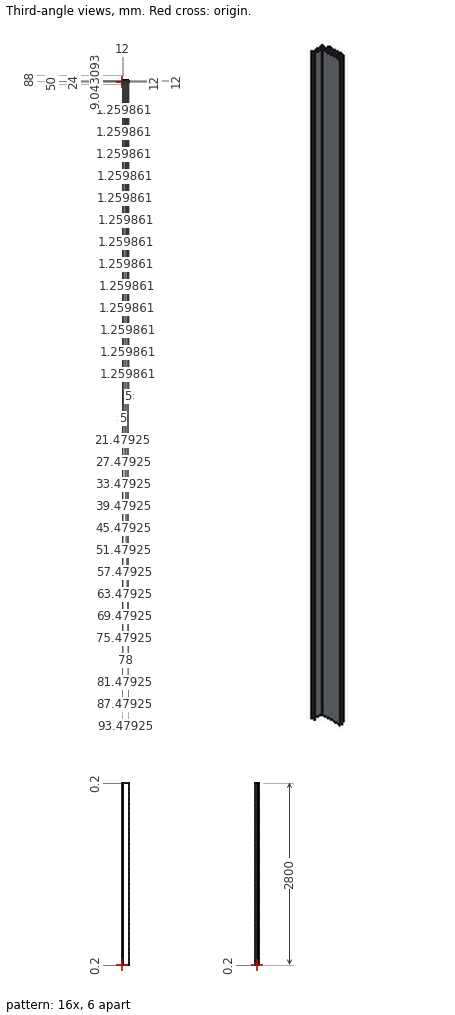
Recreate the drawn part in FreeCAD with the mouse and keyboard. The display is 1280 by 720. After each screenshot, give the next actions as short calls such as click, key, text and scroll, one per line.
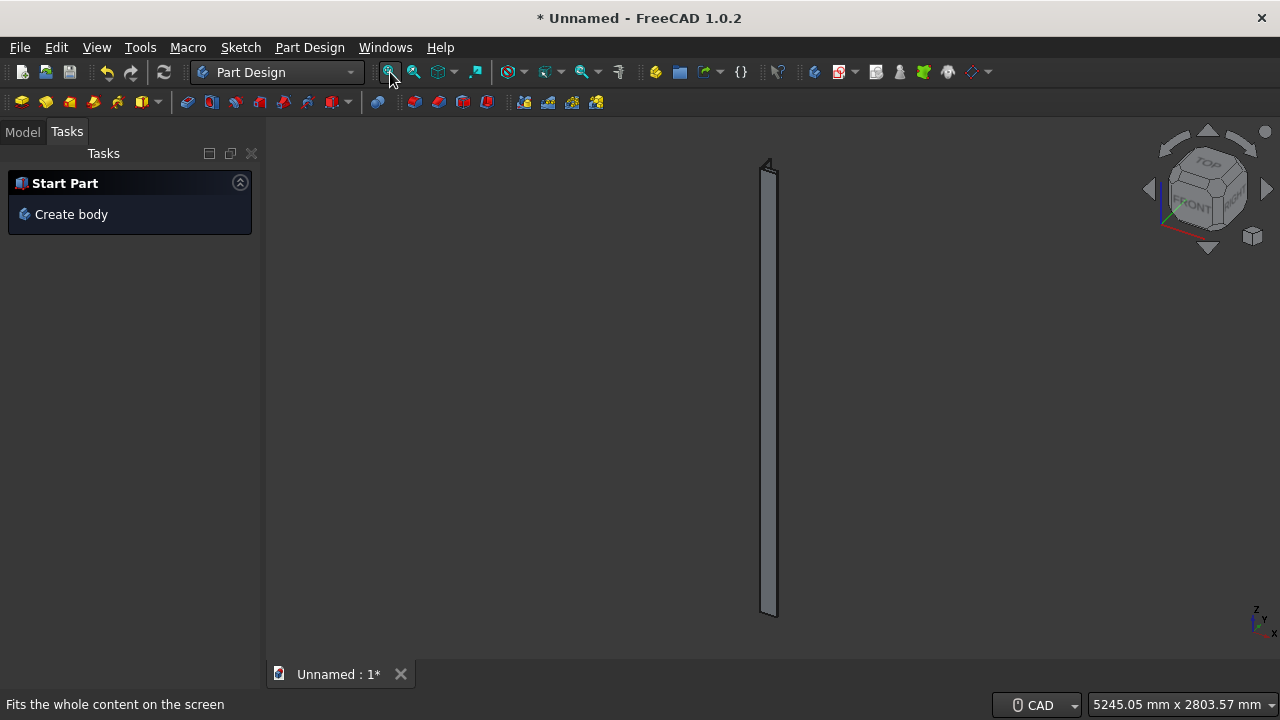
scroll(774, 171, up, 11)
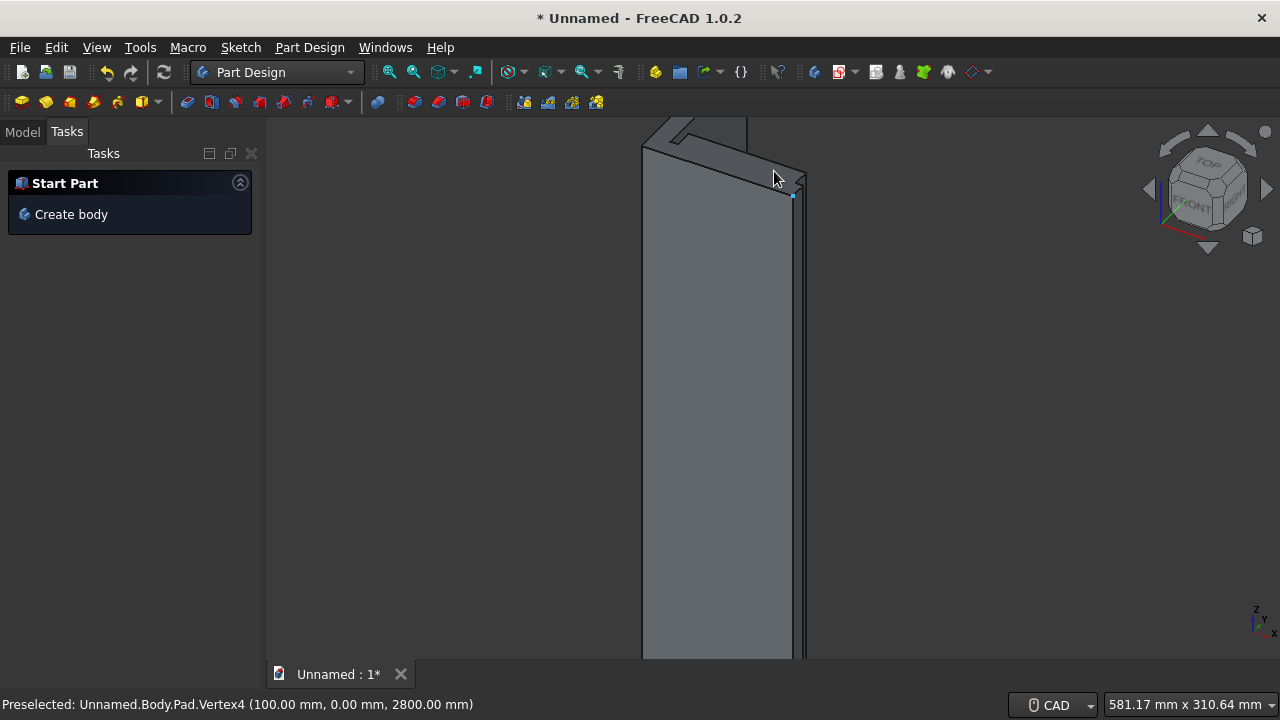
click(390, 72)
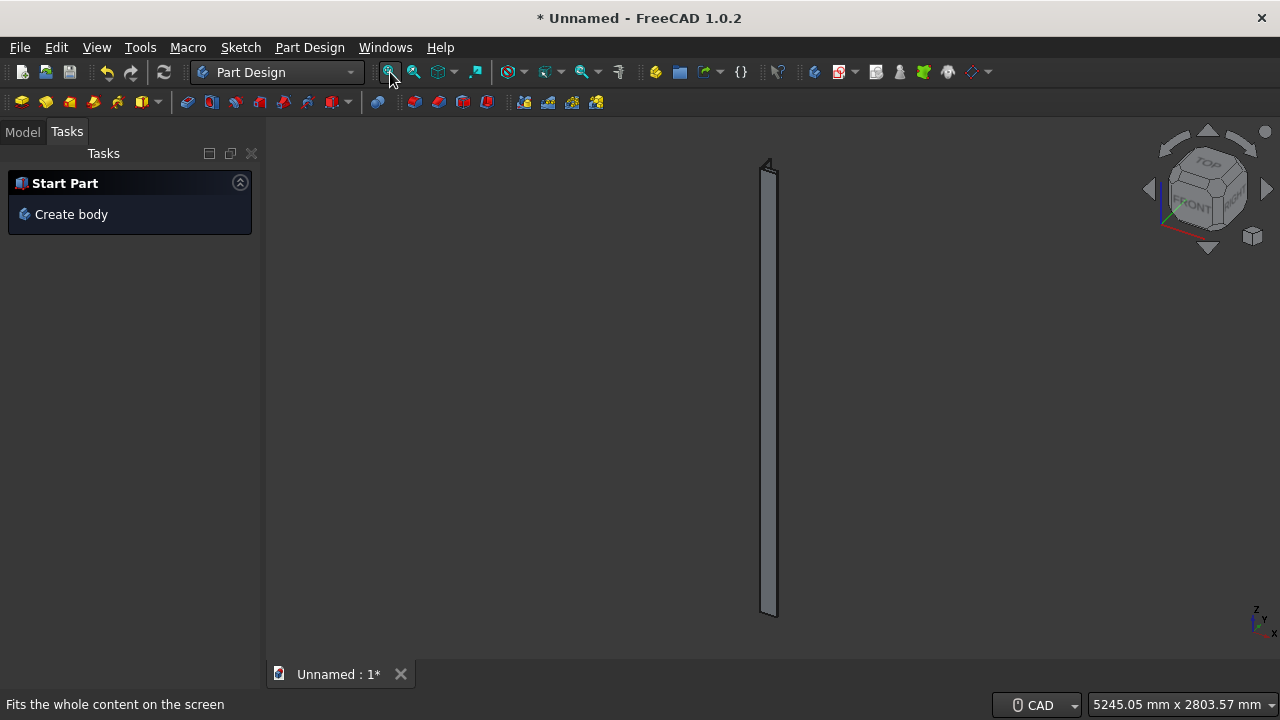
key(0)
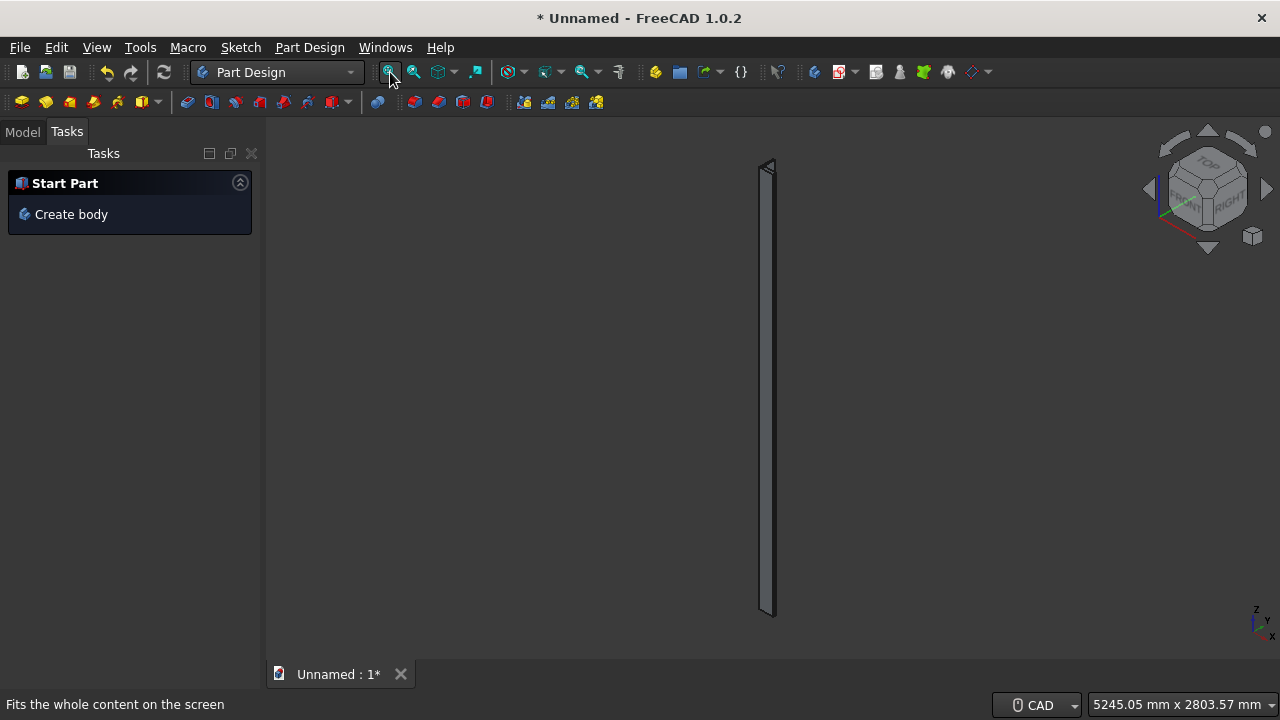
scroll(771, 172, up, 11)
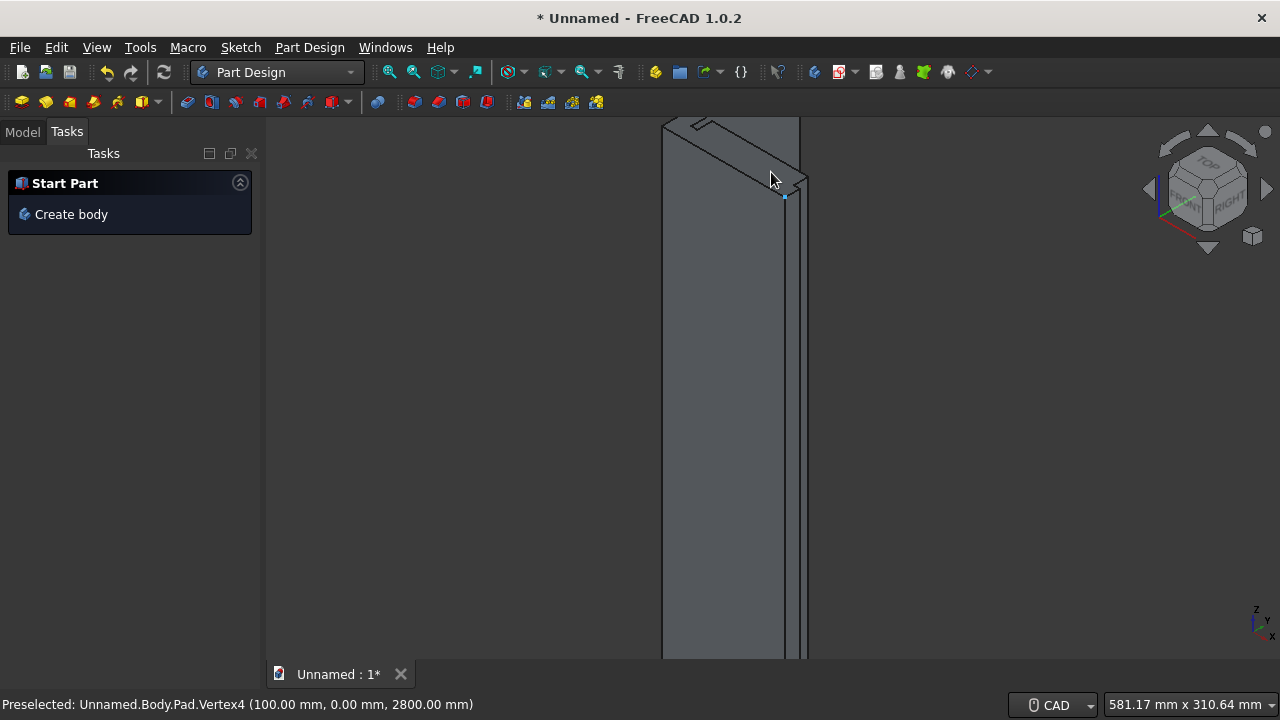
click(390, 72)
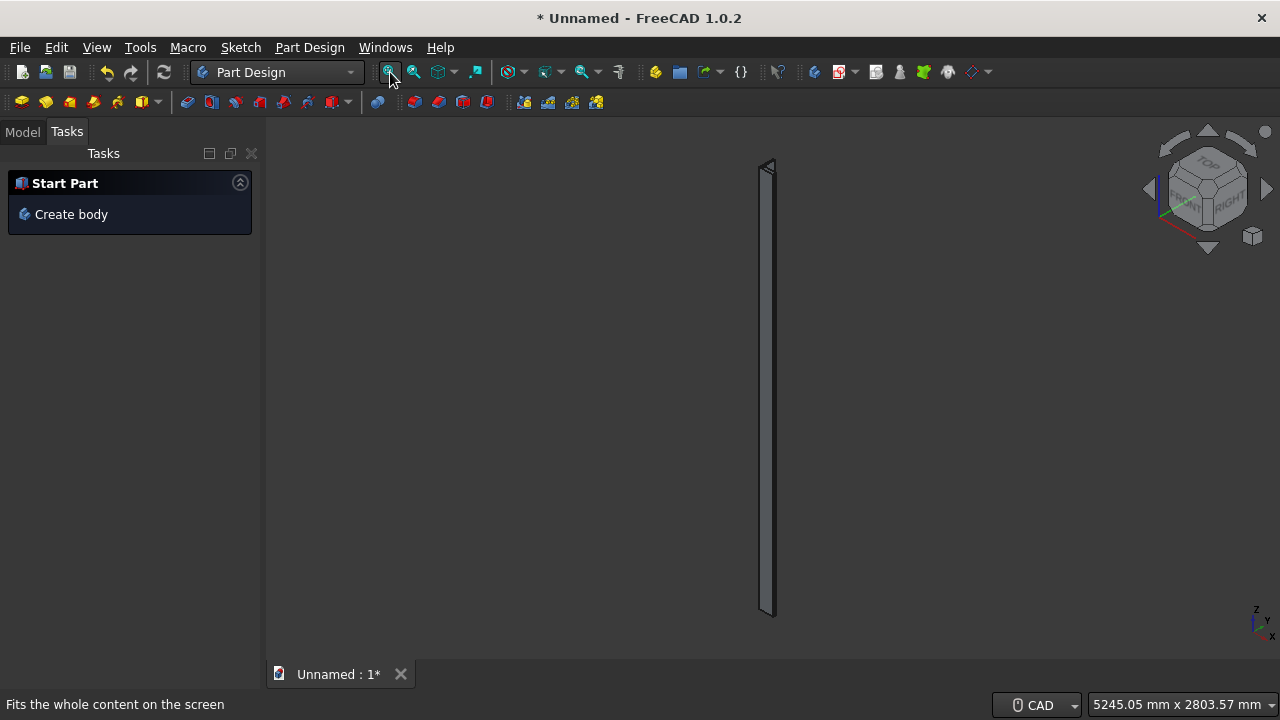
key(2)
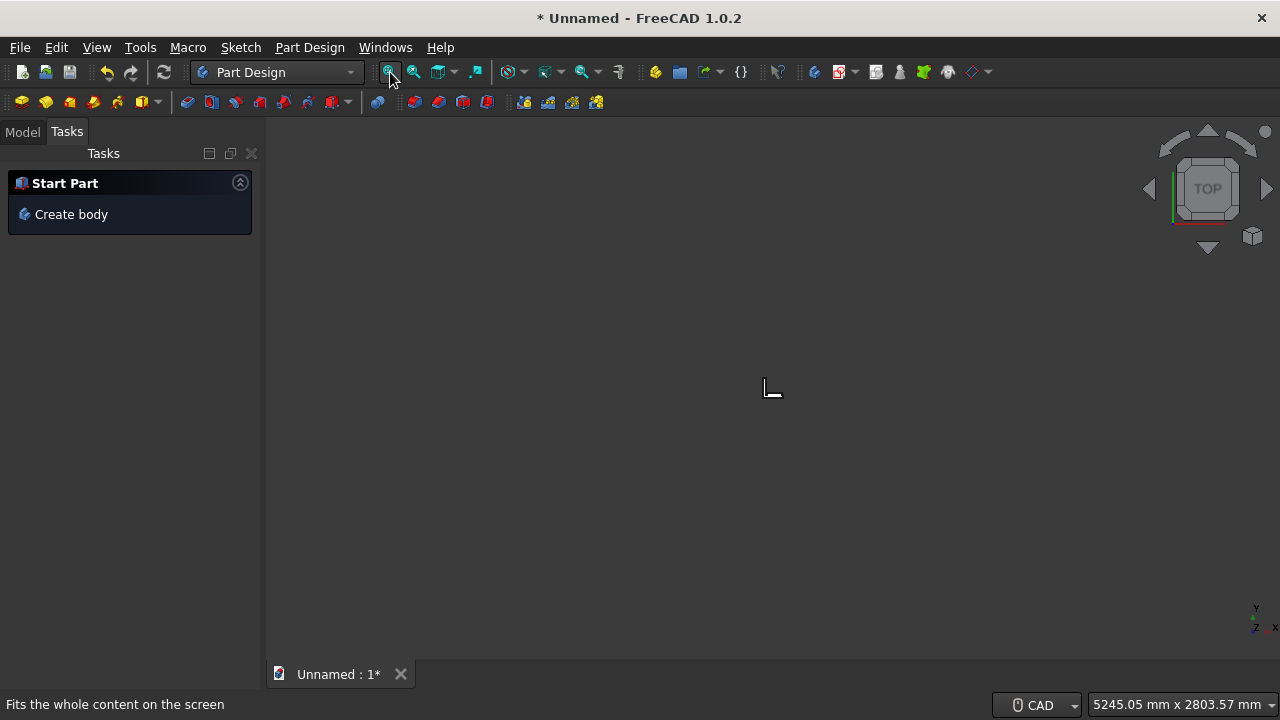
click(390, 72)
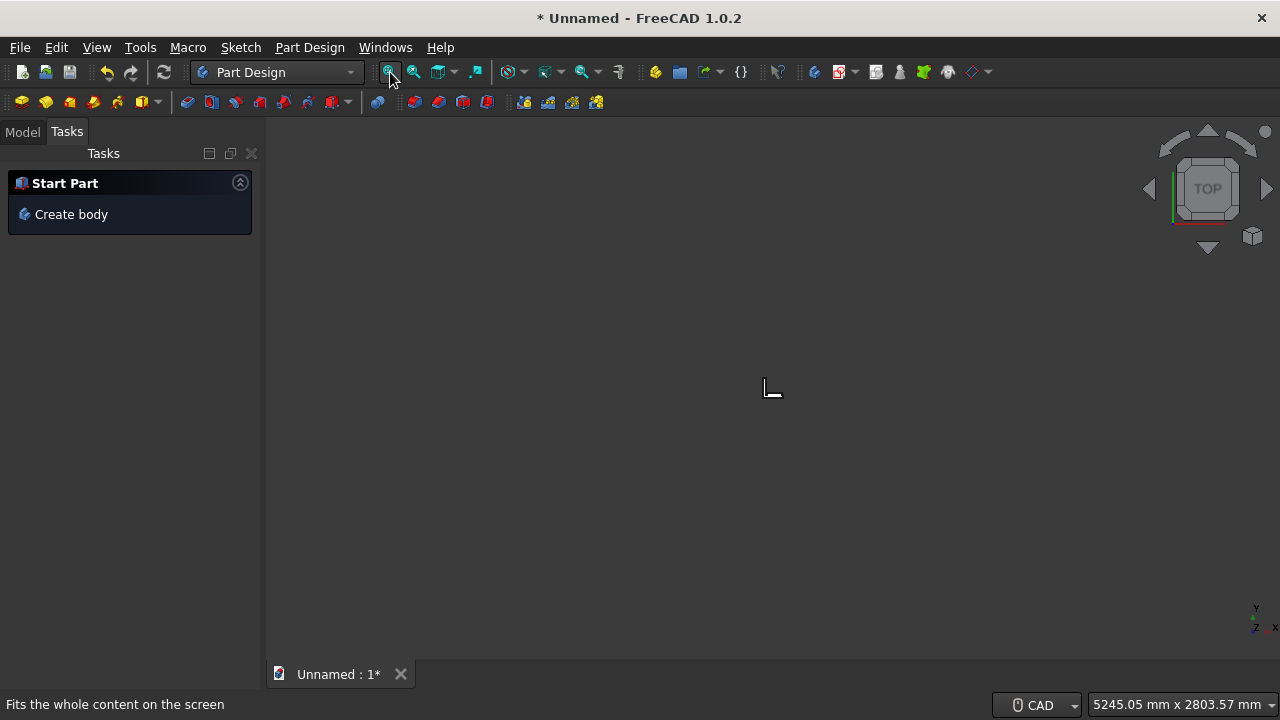
scroll(779, 395, up, 11)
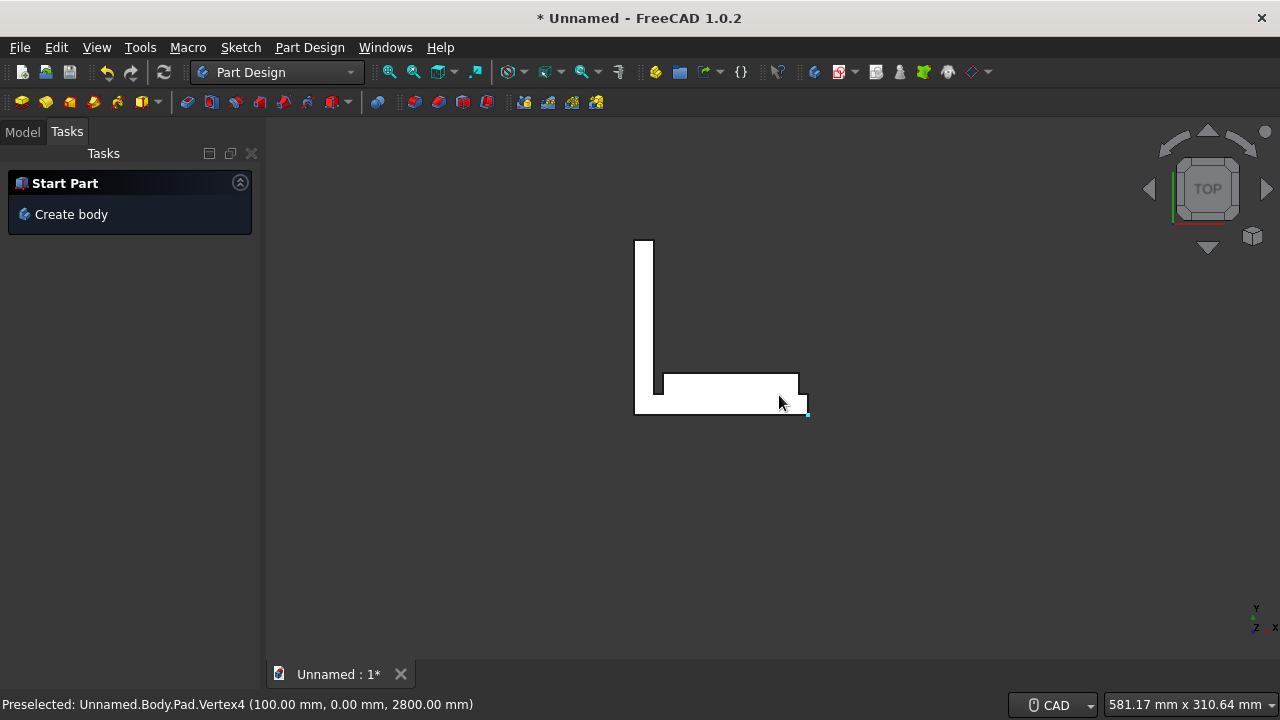
click(771, 401)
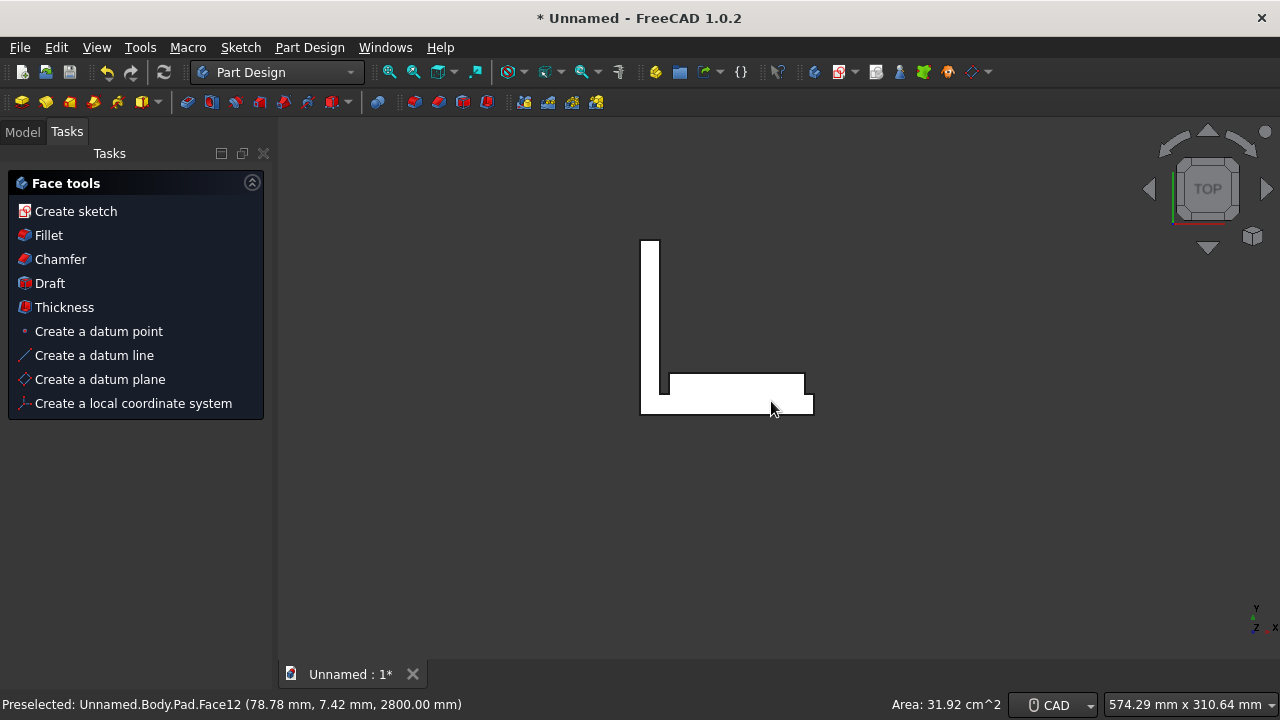
click(840, 72)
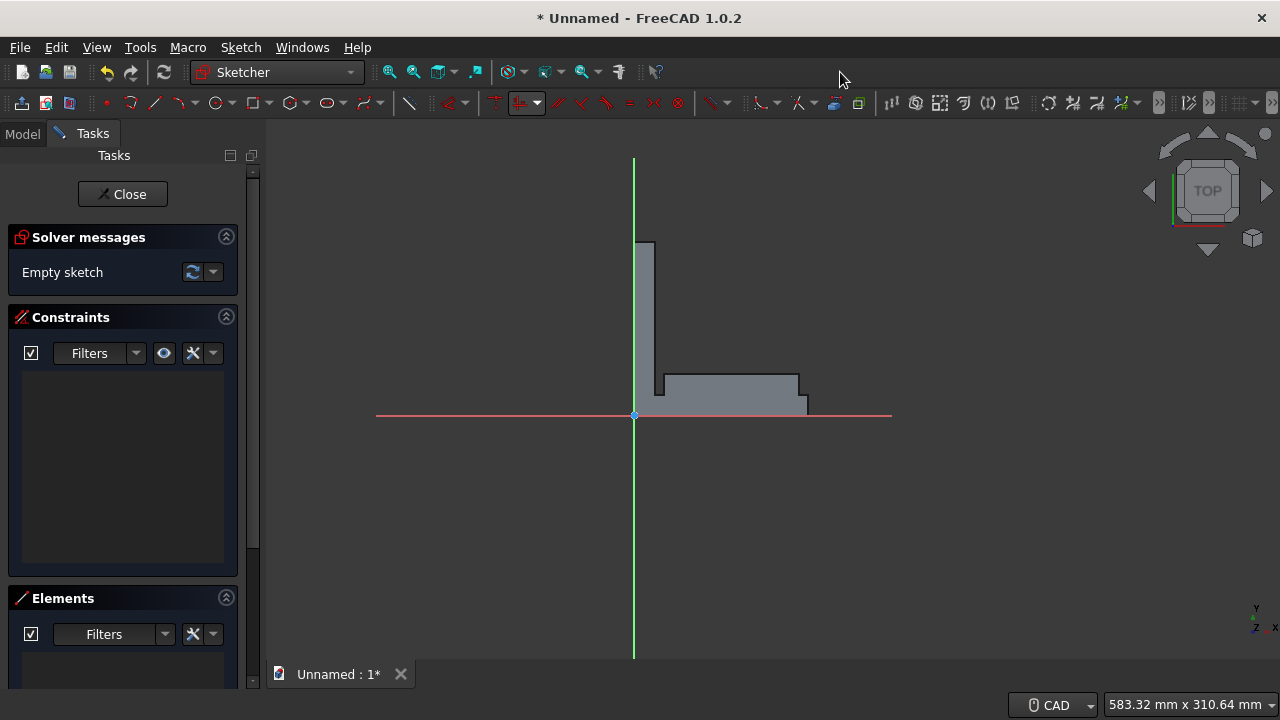
scroll(671, 382, up, 15)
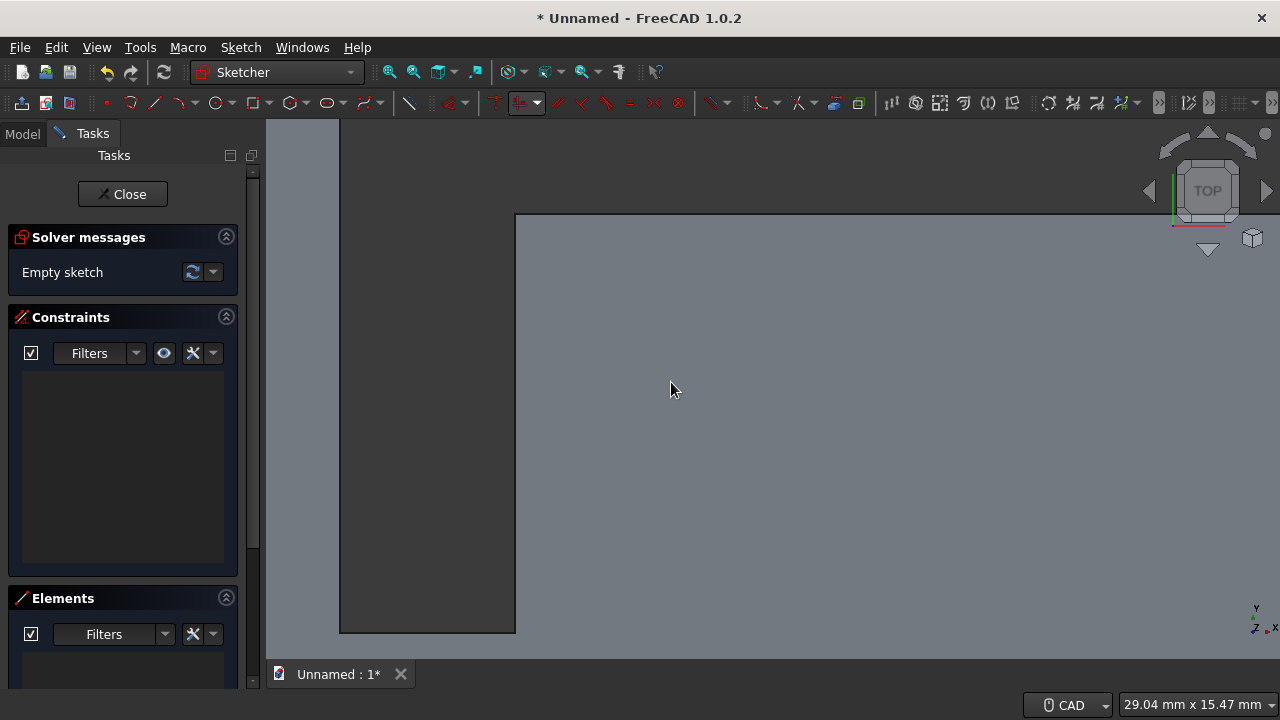
click(254, 104)